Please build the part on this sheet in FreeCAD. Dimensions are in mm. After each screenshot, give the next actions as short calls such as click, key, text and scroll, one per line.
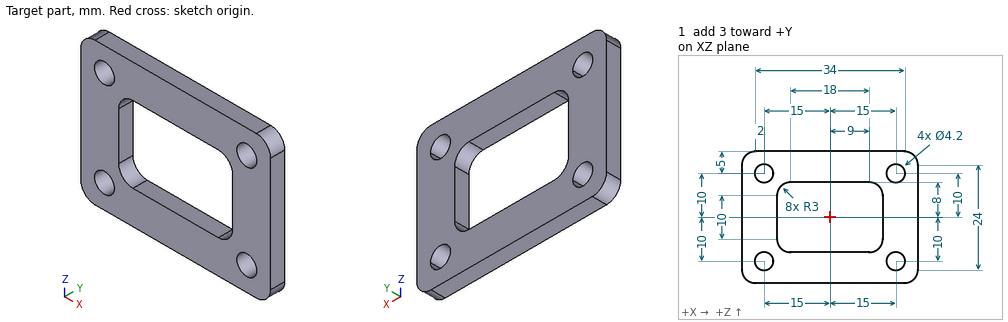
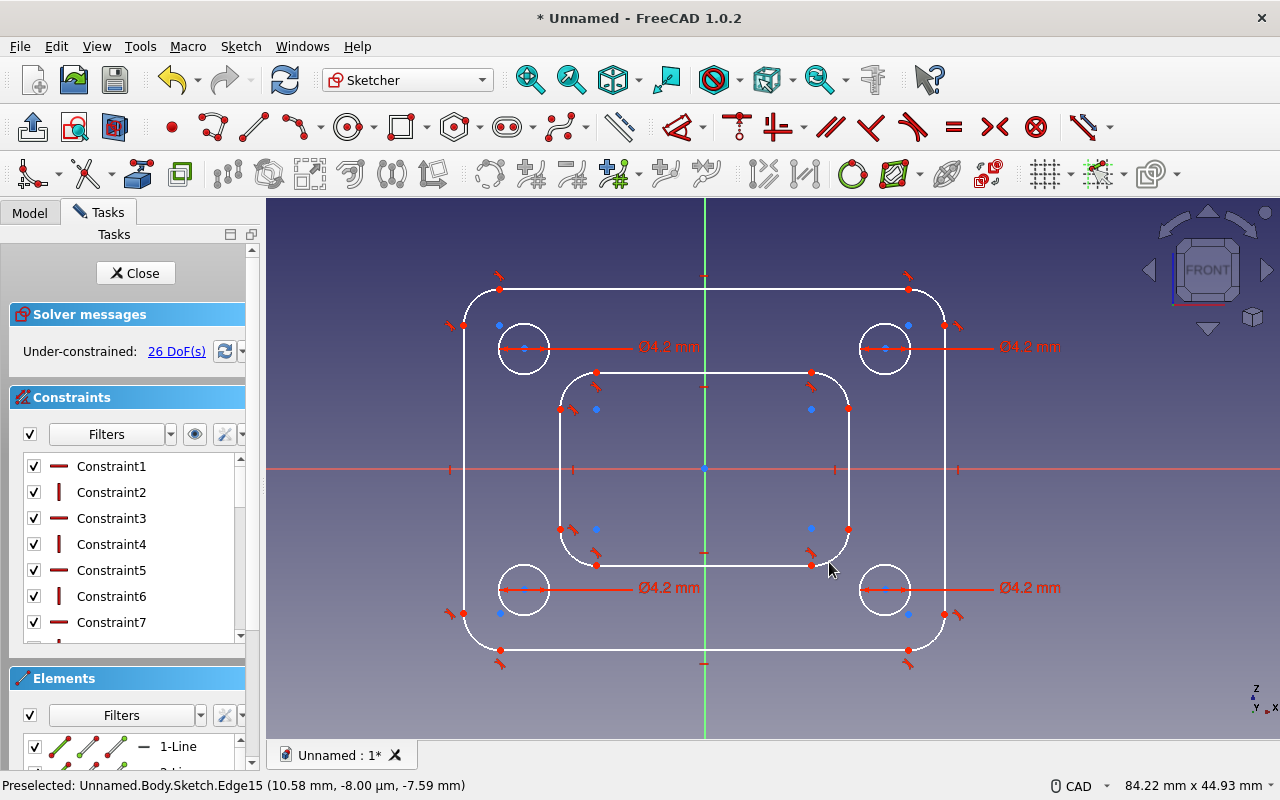
click(849, 494)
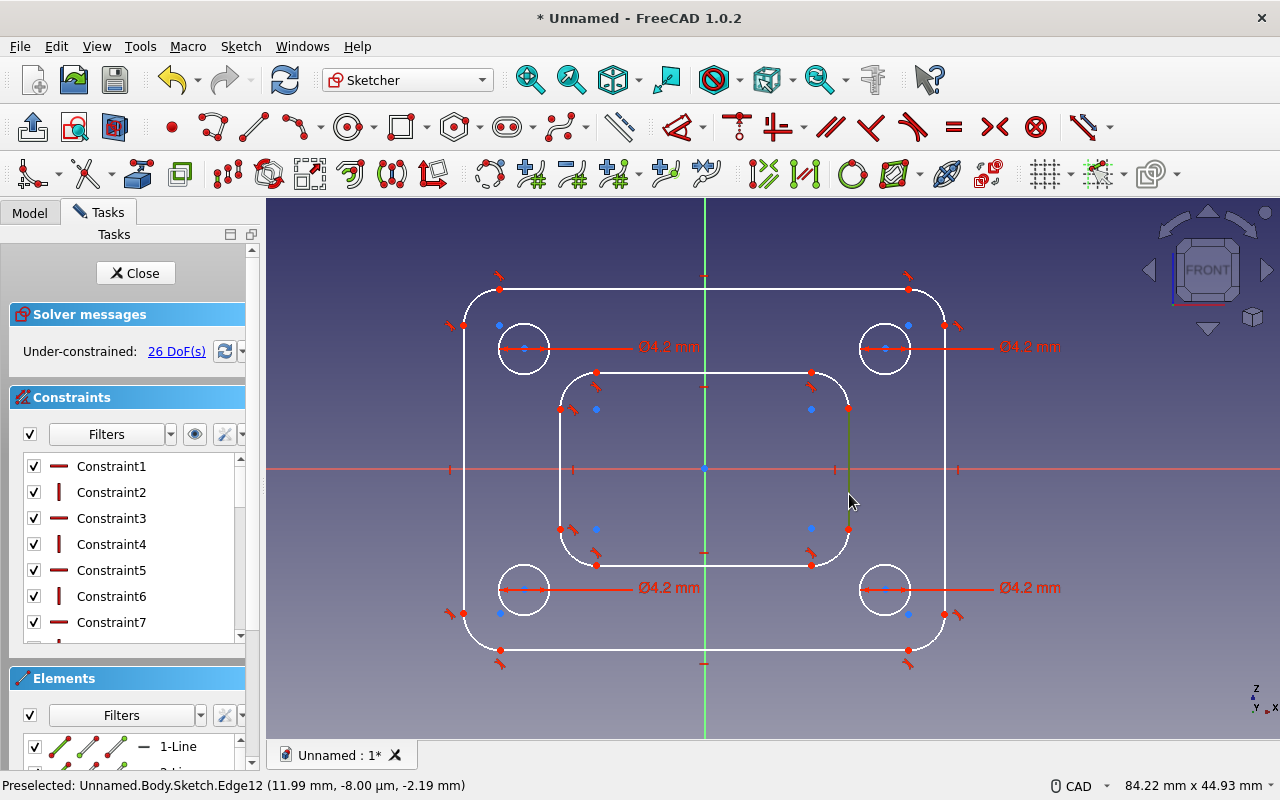
click(828, 562)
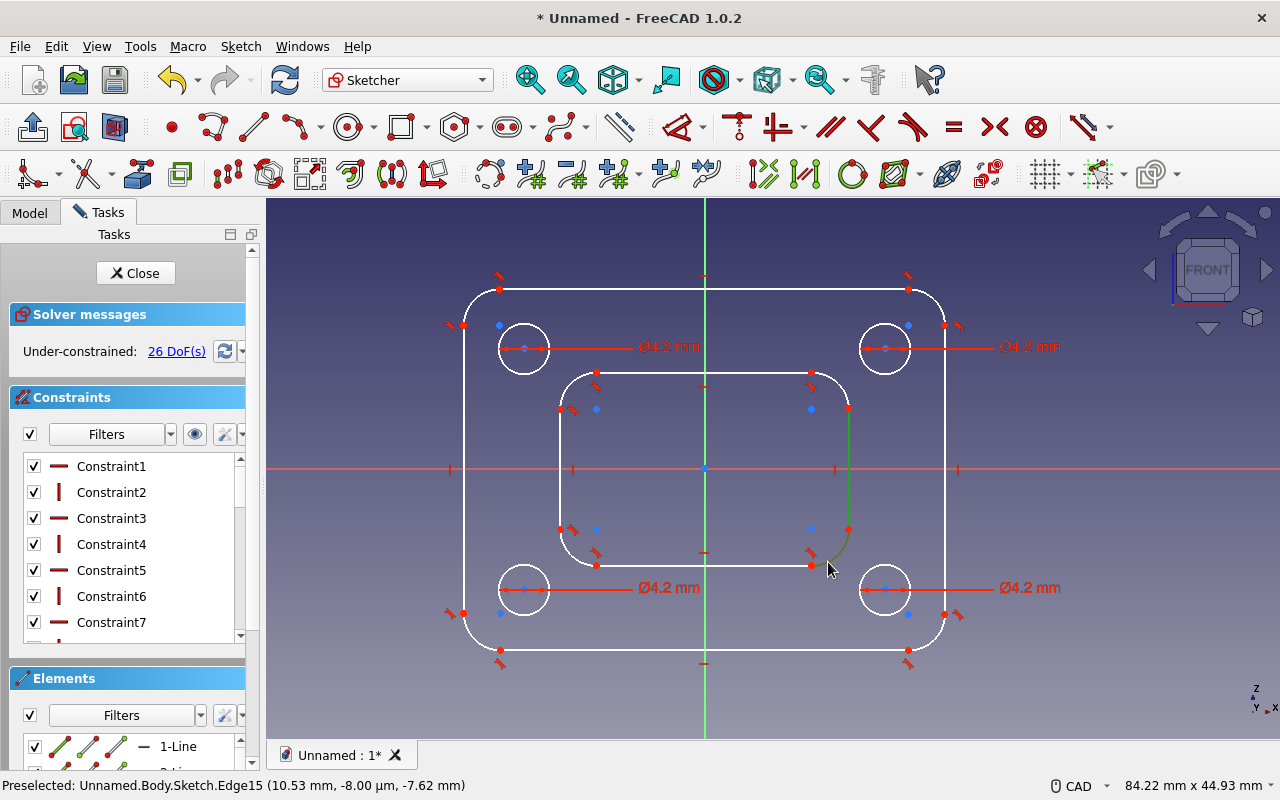
key(t)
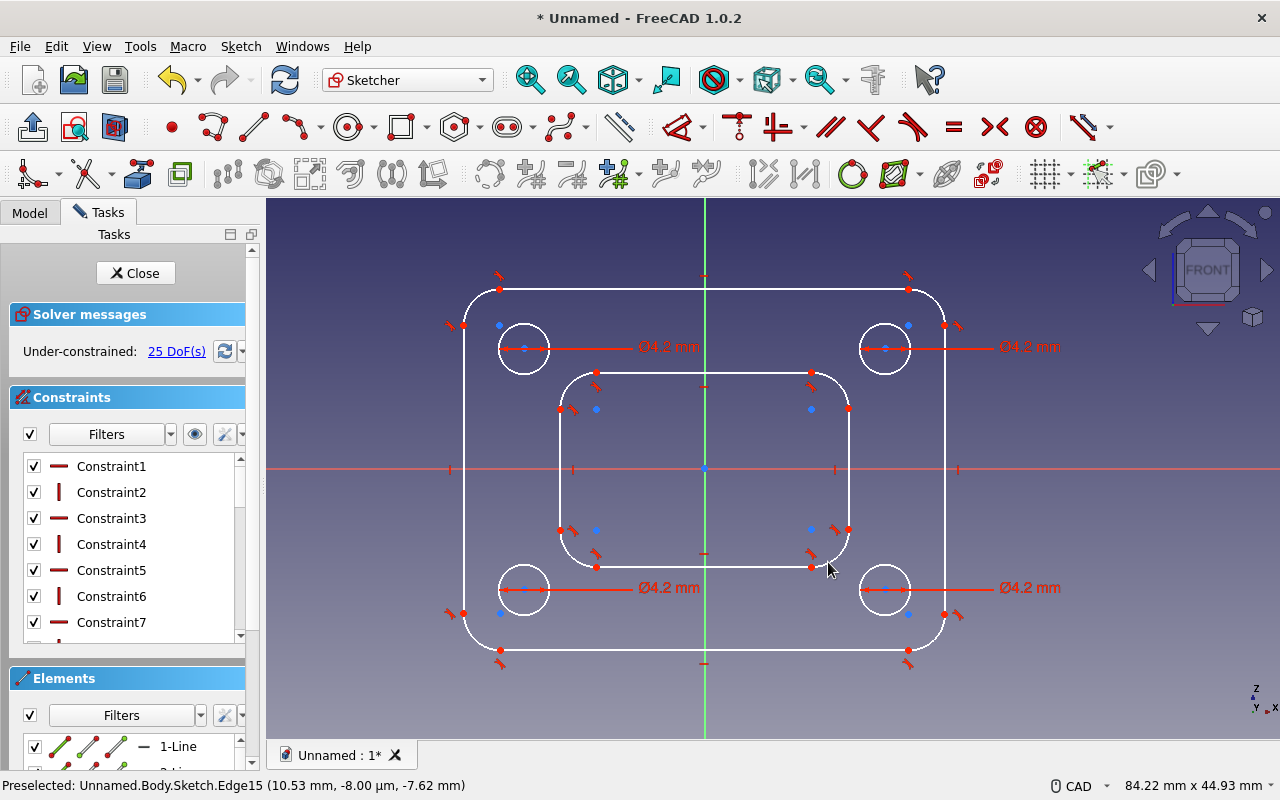
click(849, 494)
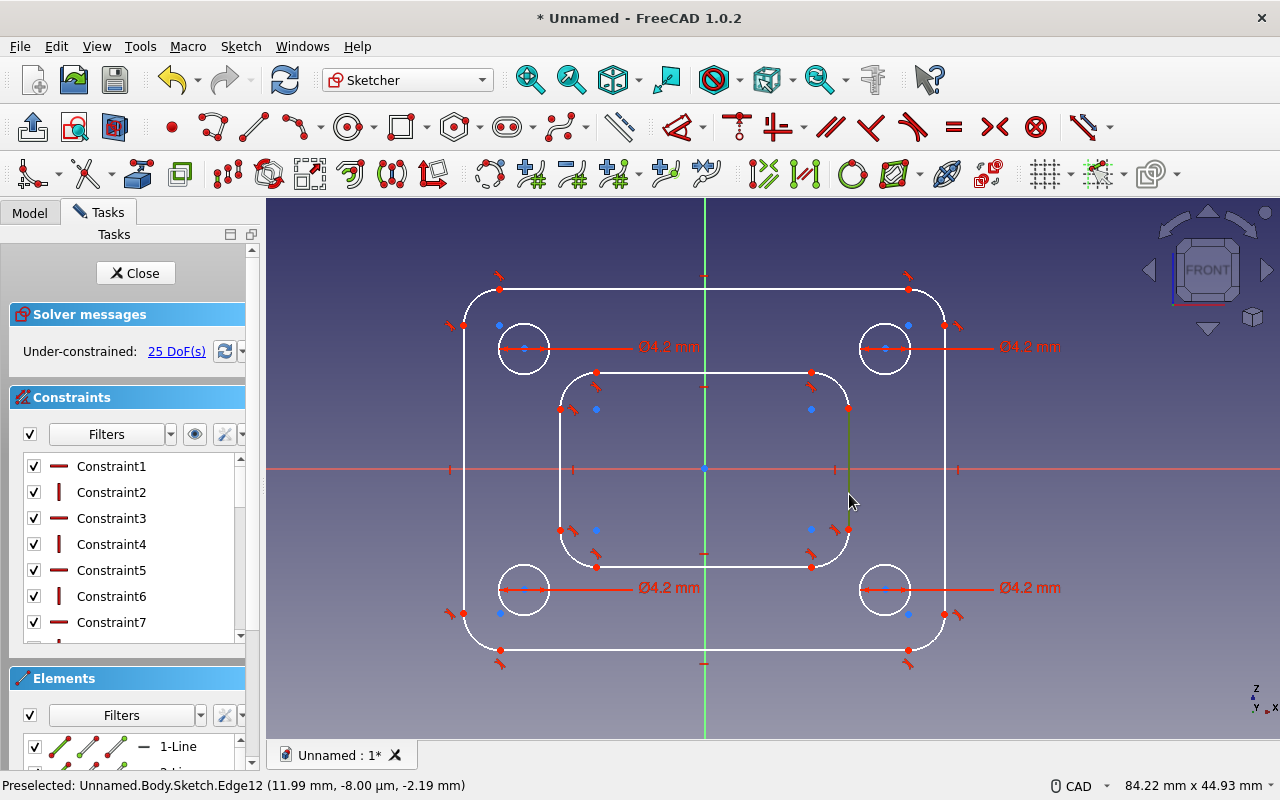
click(845, 392)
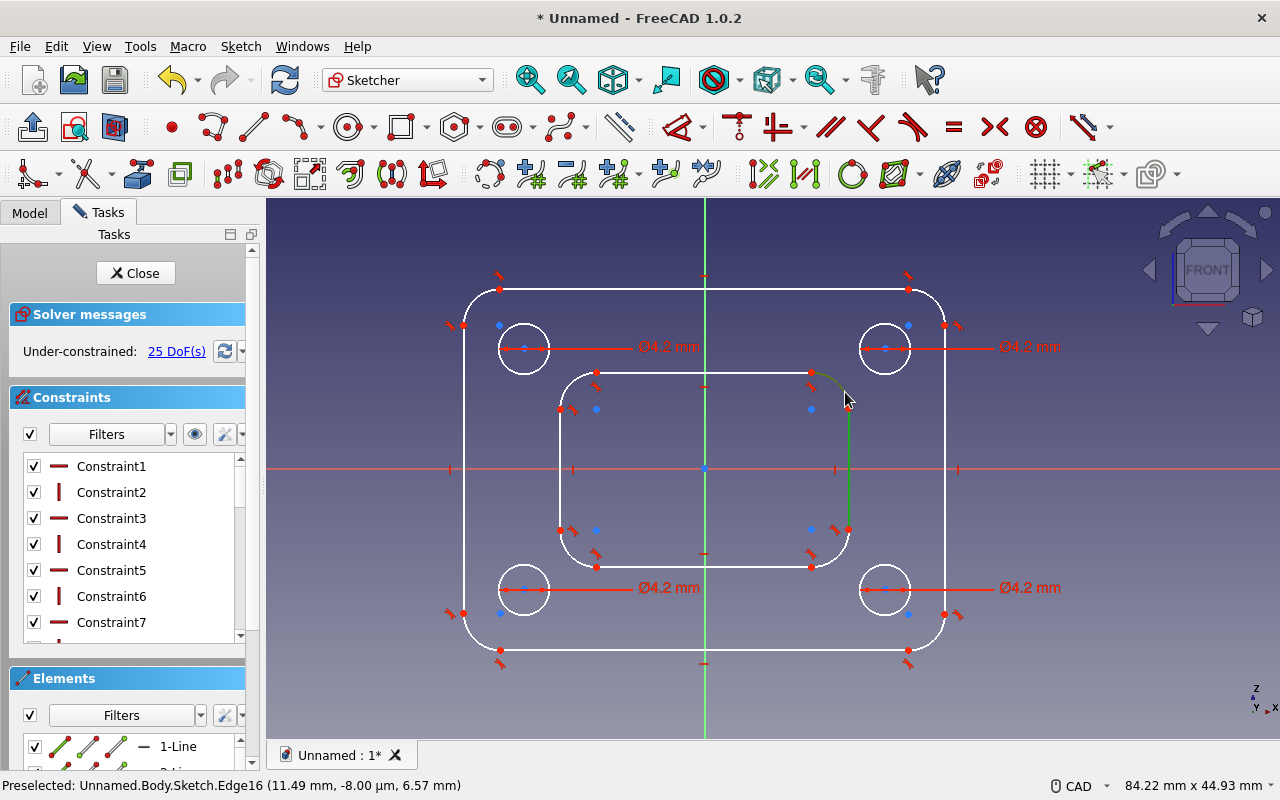
click(913, 128)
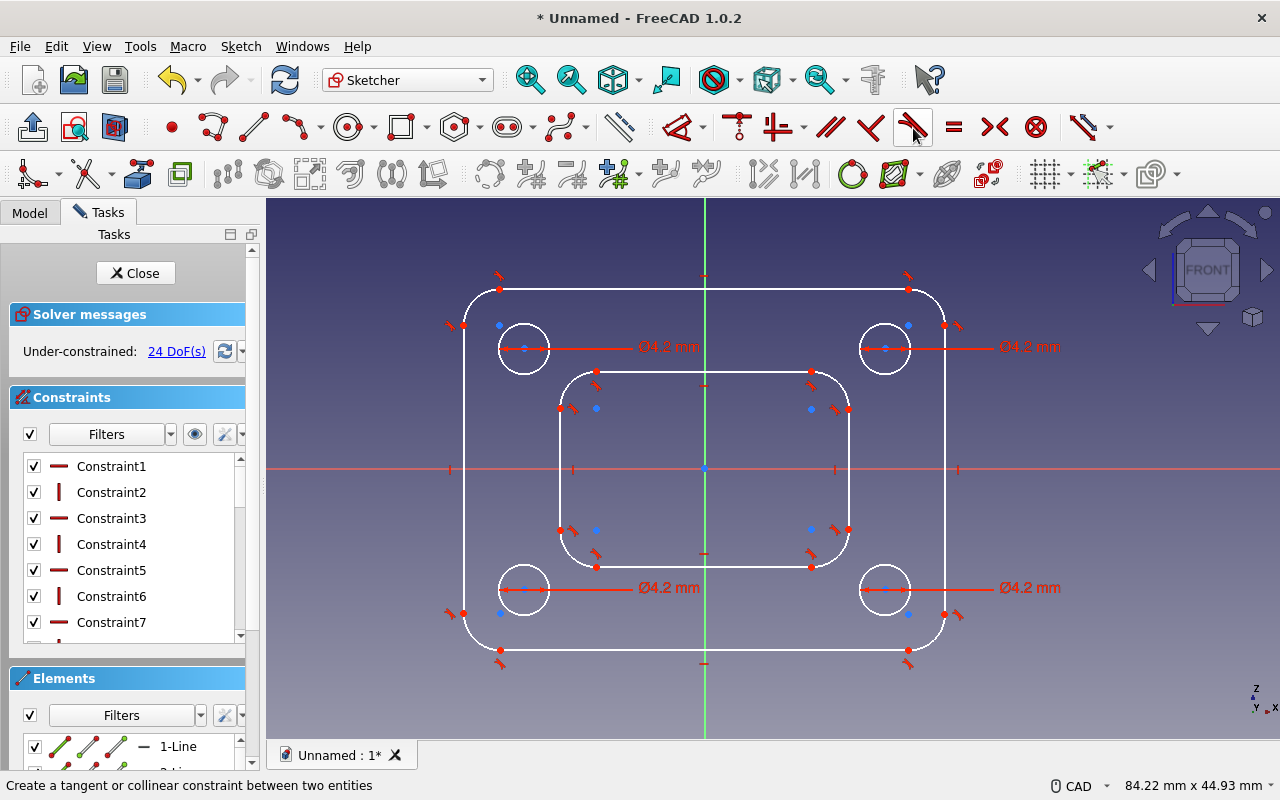
click(941, 309)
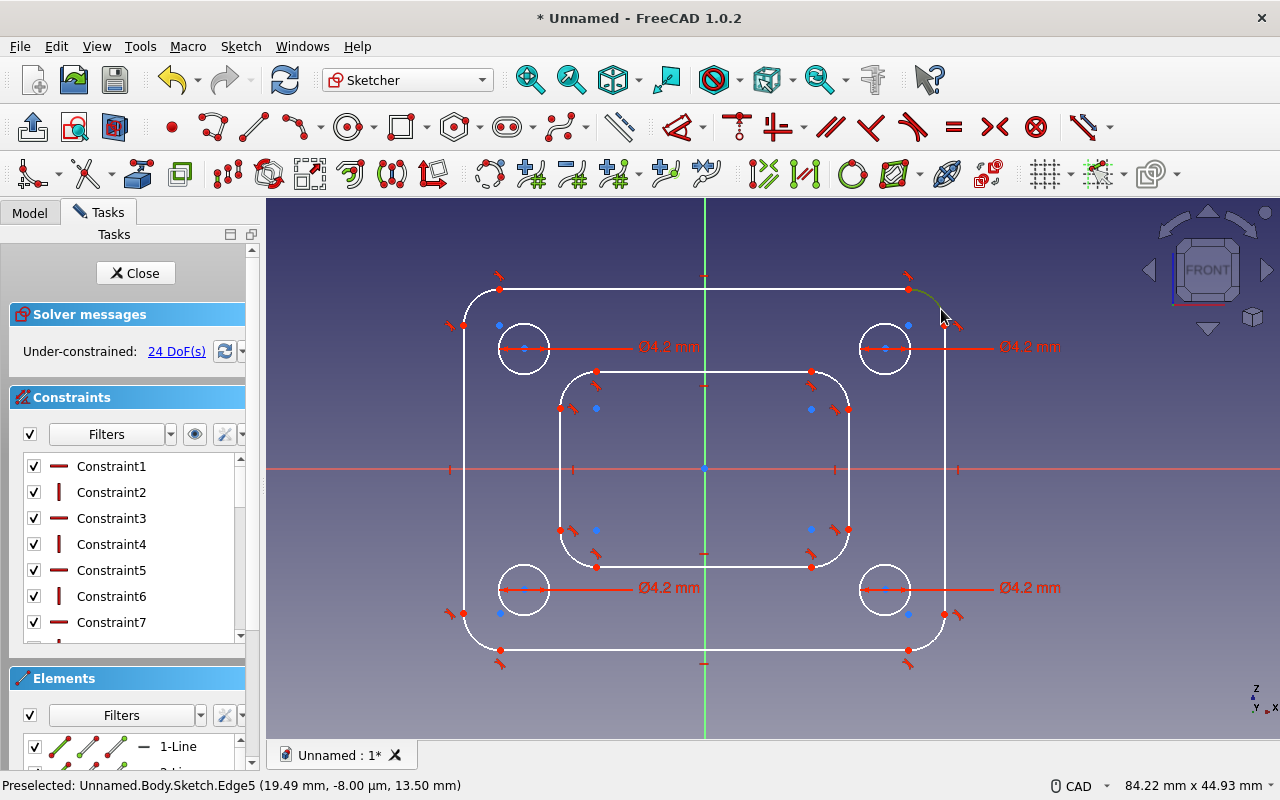
click(925, 646)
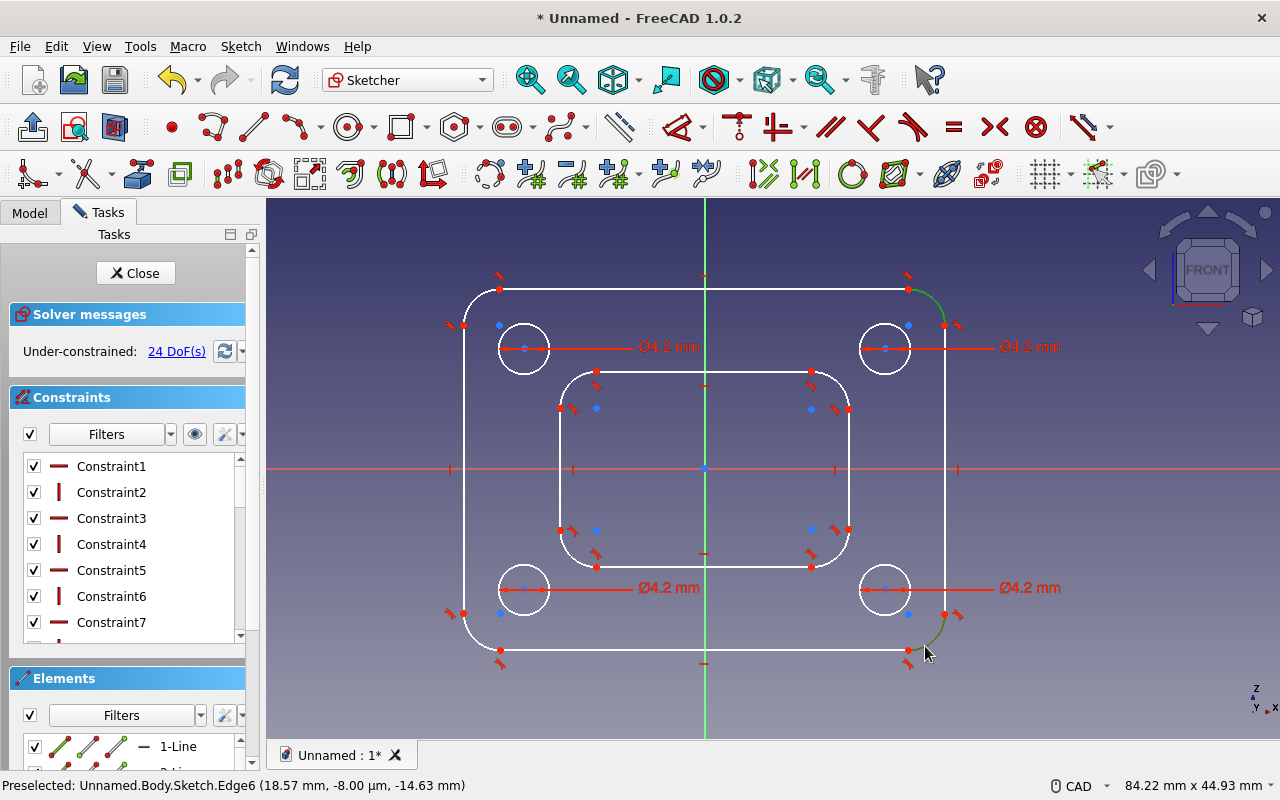
click(468, 630)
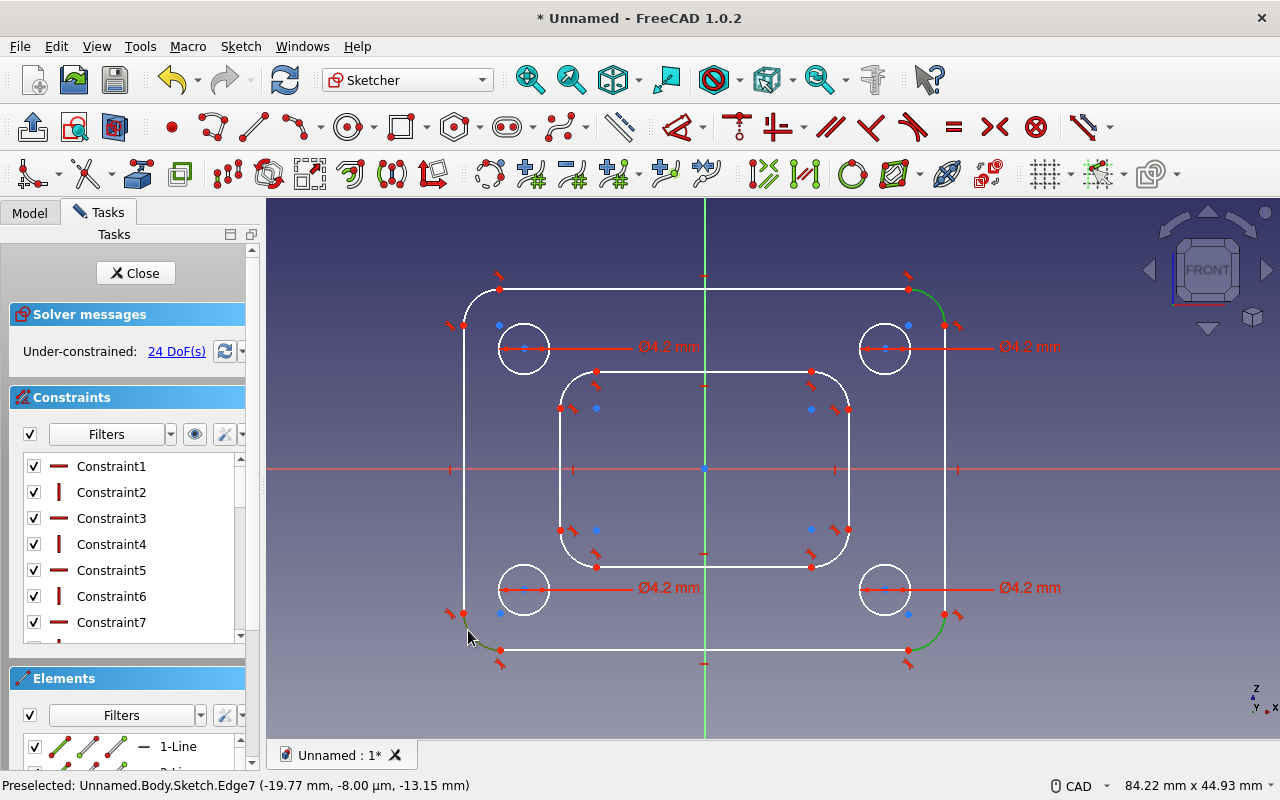
click(484, 293)